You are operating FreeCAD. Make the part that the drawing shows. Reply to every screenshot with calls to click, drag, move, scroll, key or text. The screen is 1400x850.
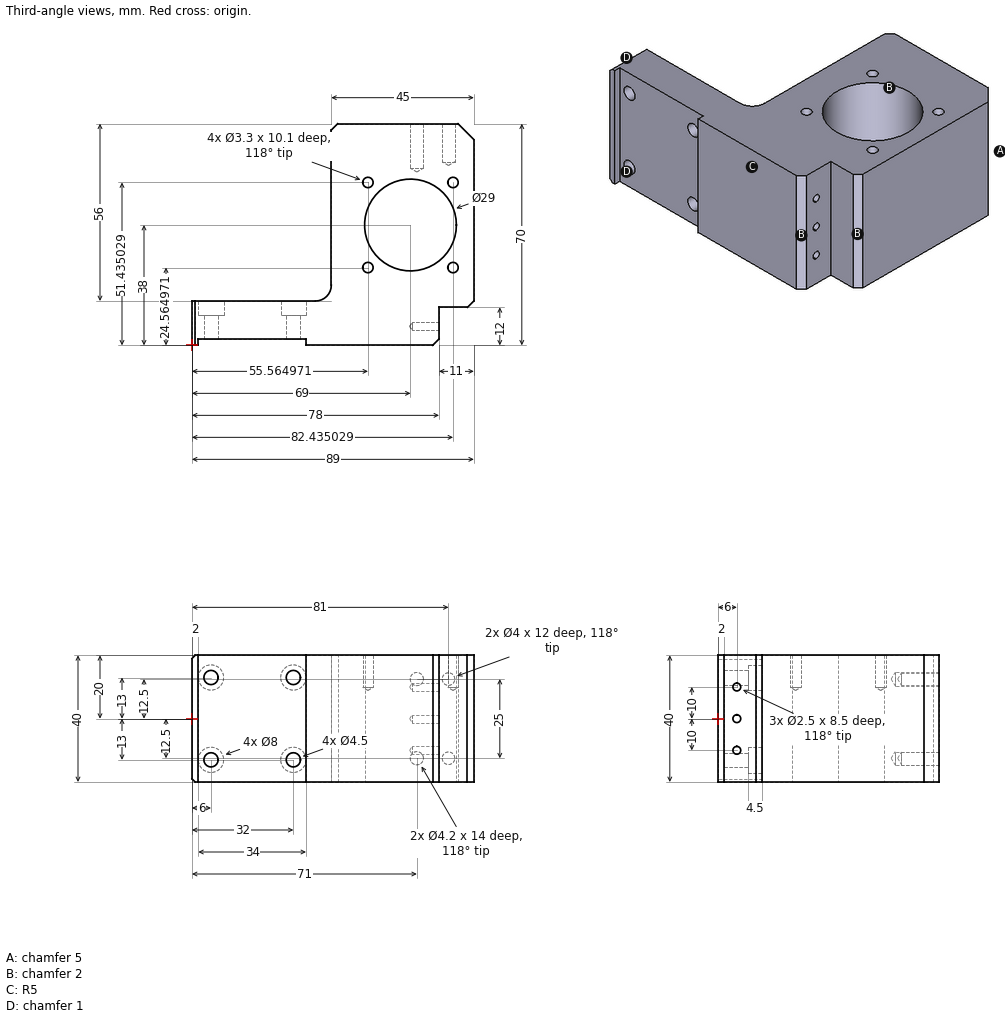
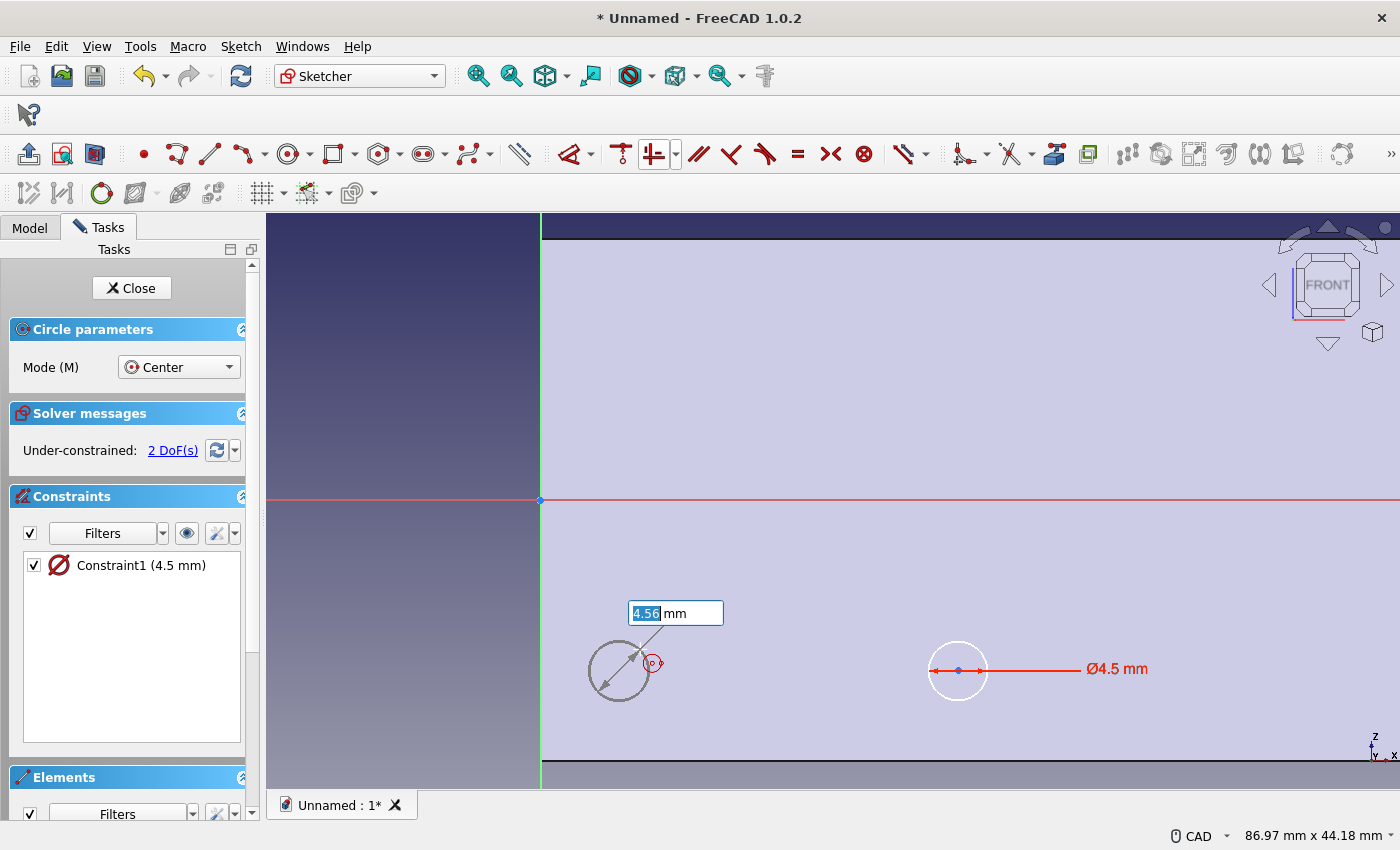
text(4.5)
key(Return)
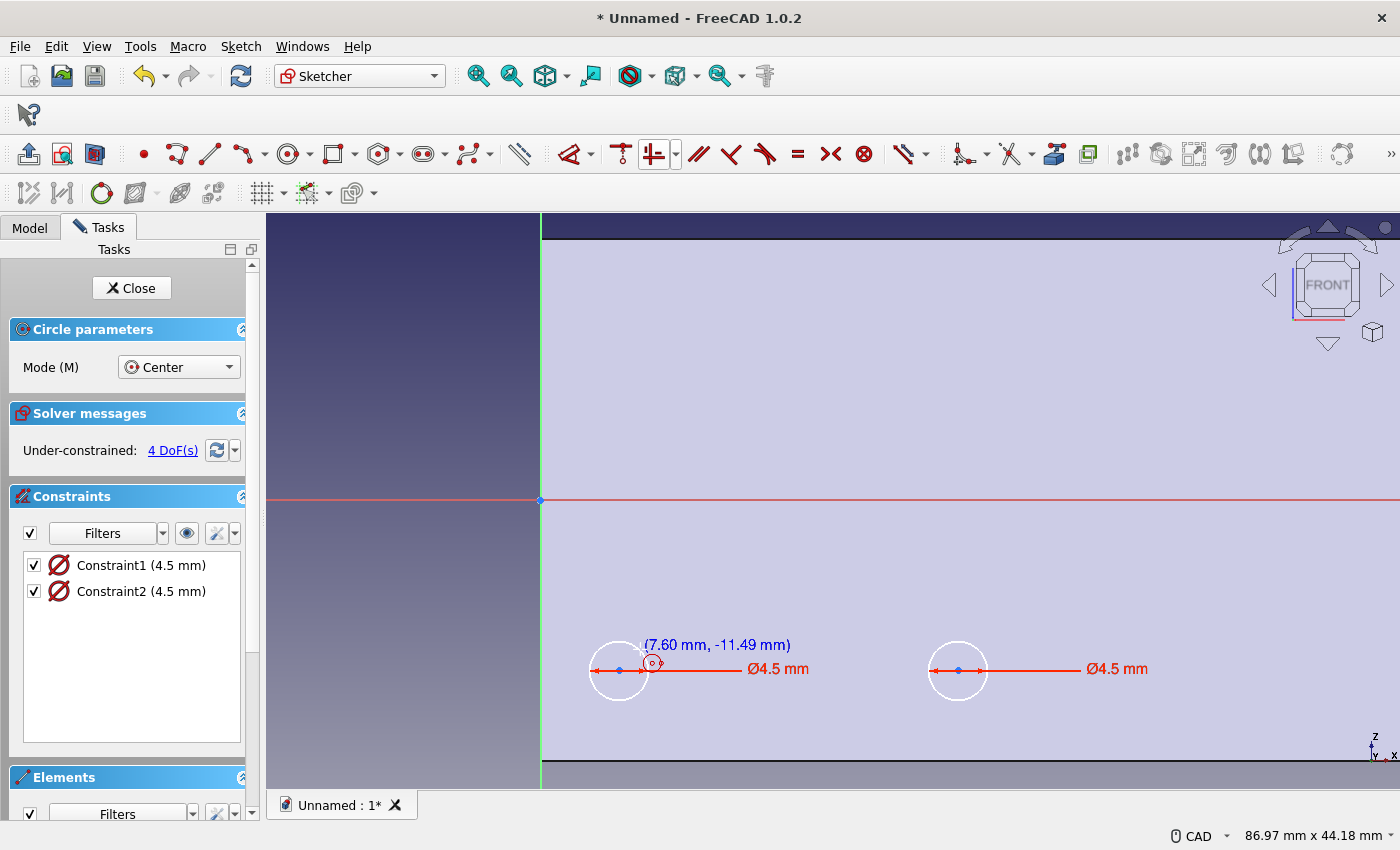
click(619, 331)
move(640, 310)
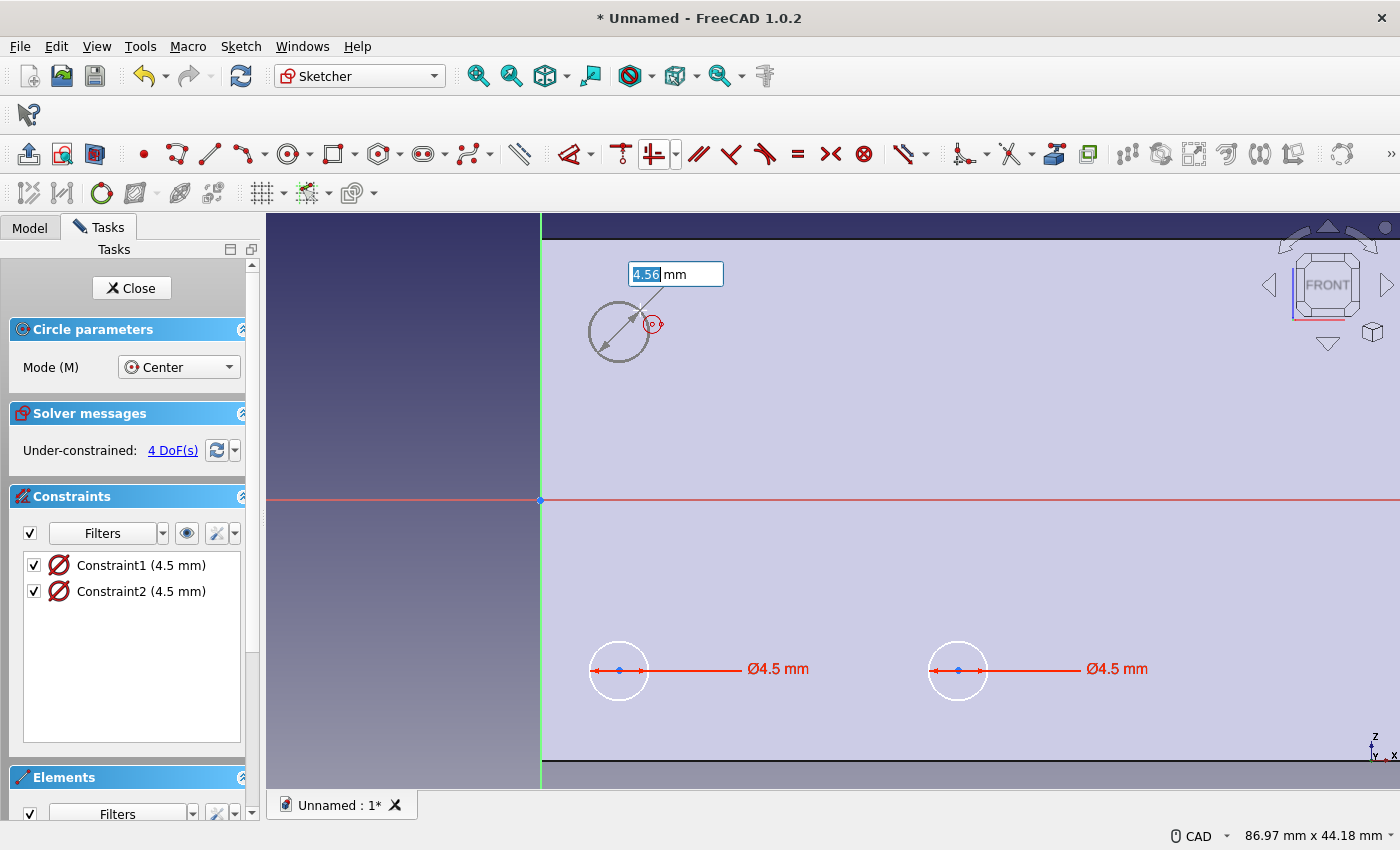
text(4.5)
key(Return)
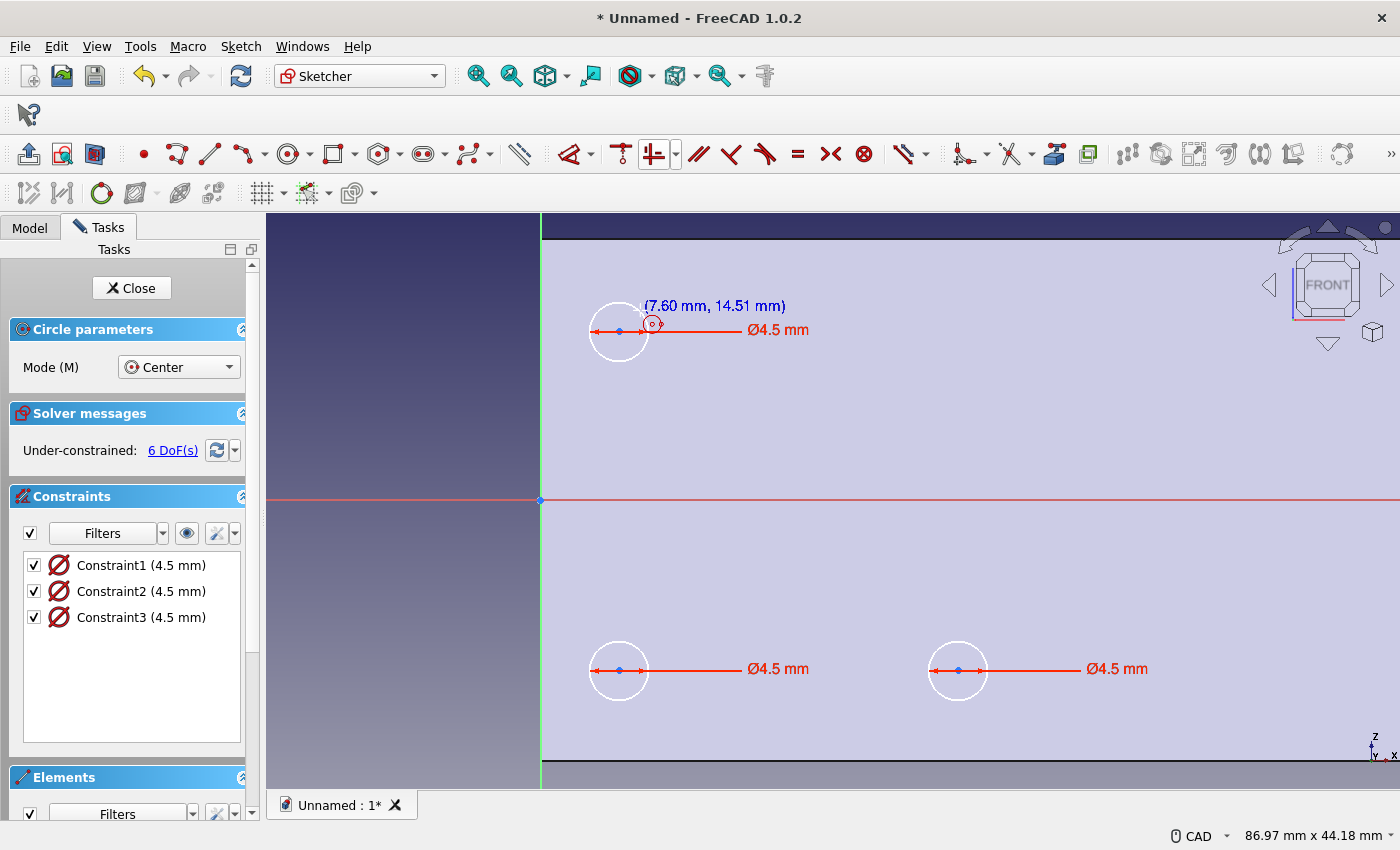
click(958, 331)
move(979, 310)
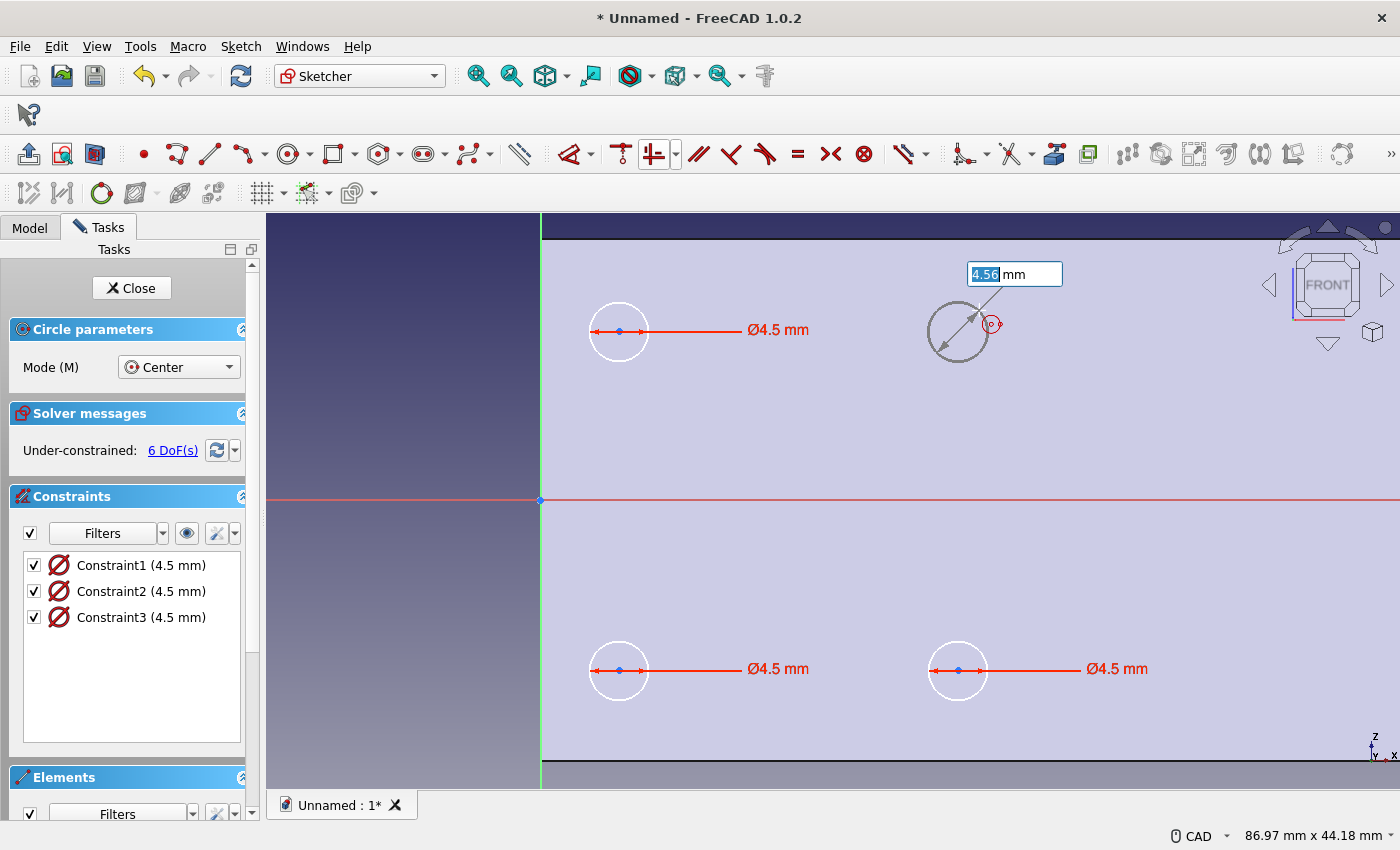
text(4.5)
key(Return)
key(Escape)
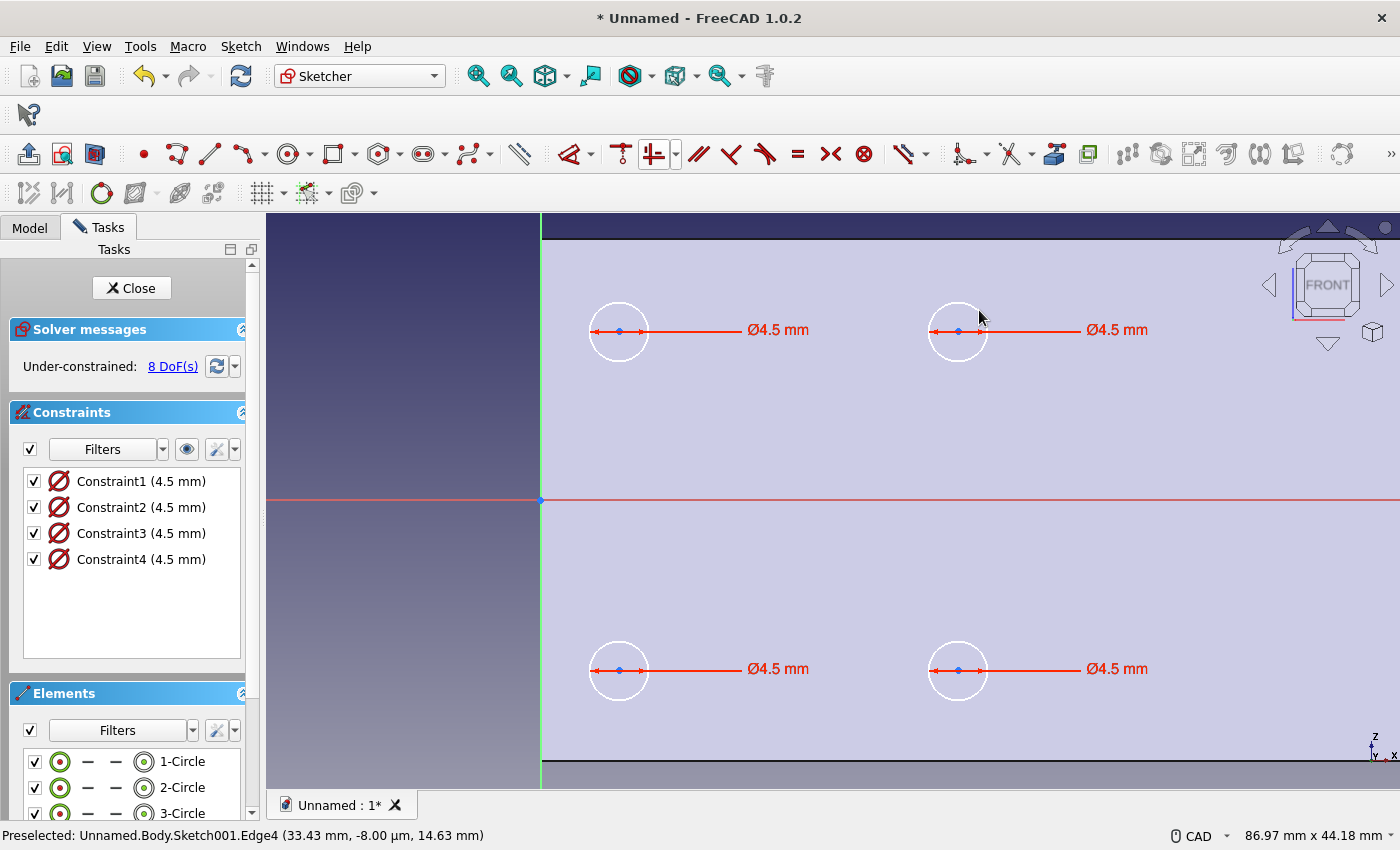
click(958, 671)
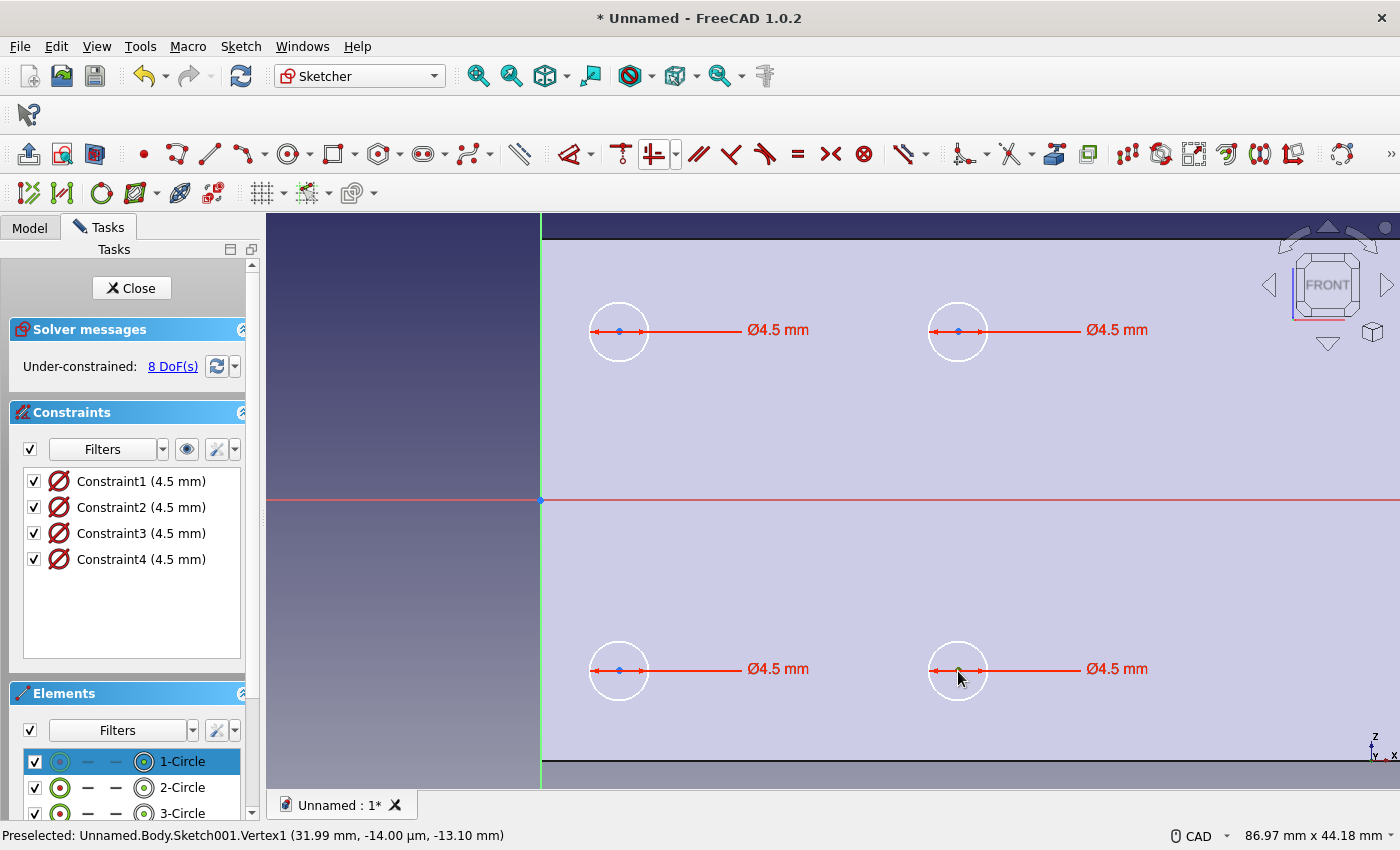
click(619, 671)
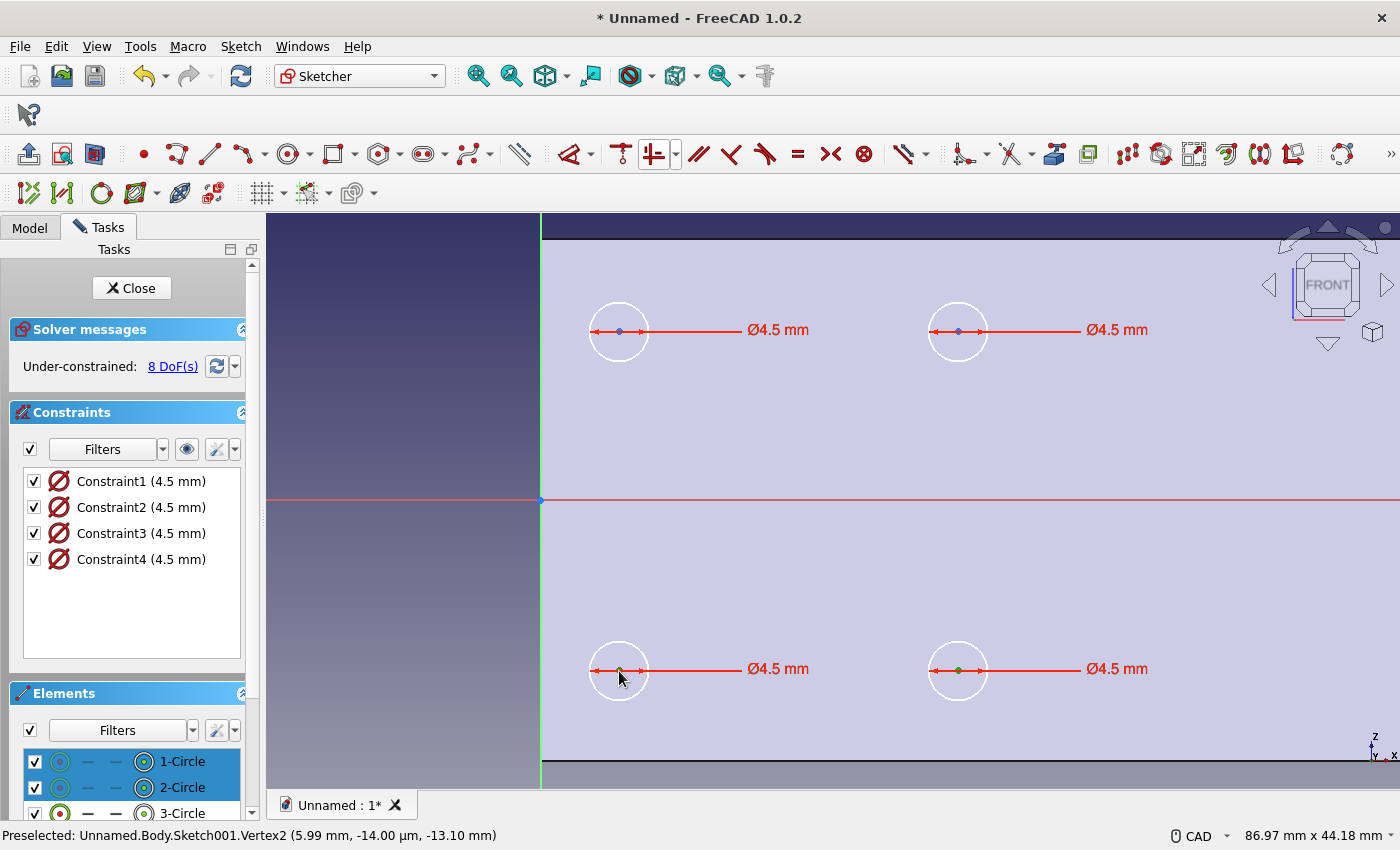
key(h)